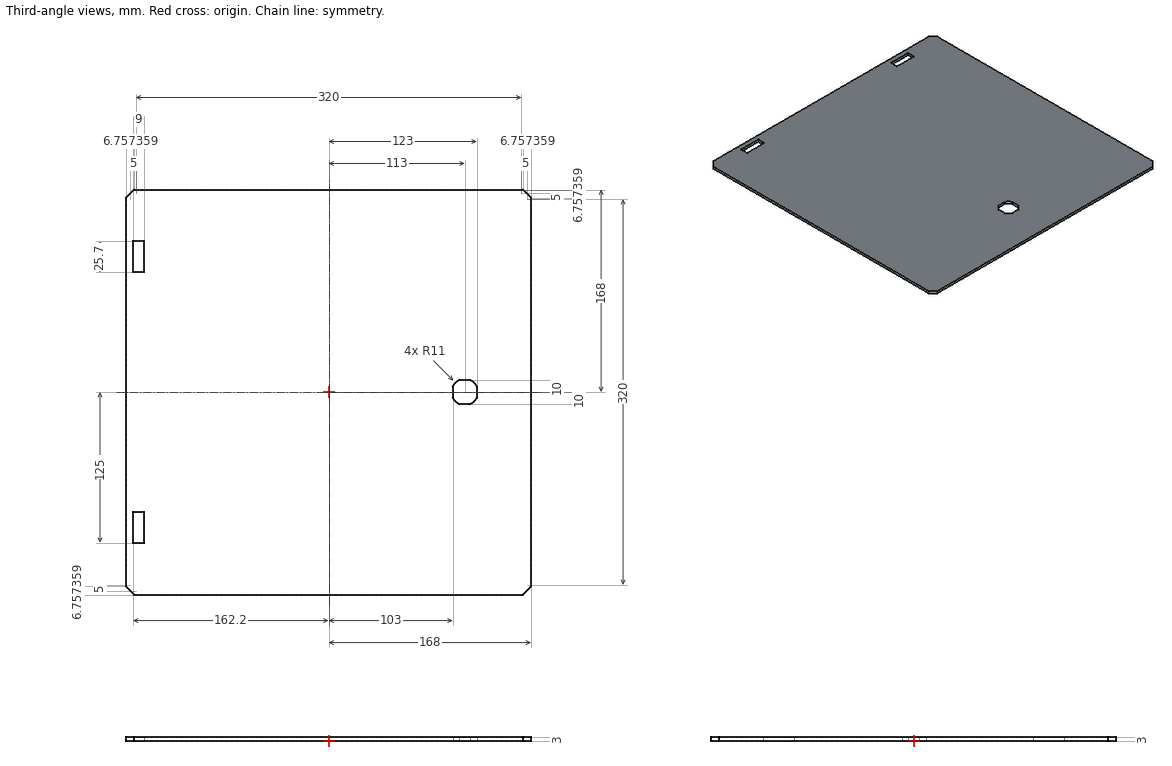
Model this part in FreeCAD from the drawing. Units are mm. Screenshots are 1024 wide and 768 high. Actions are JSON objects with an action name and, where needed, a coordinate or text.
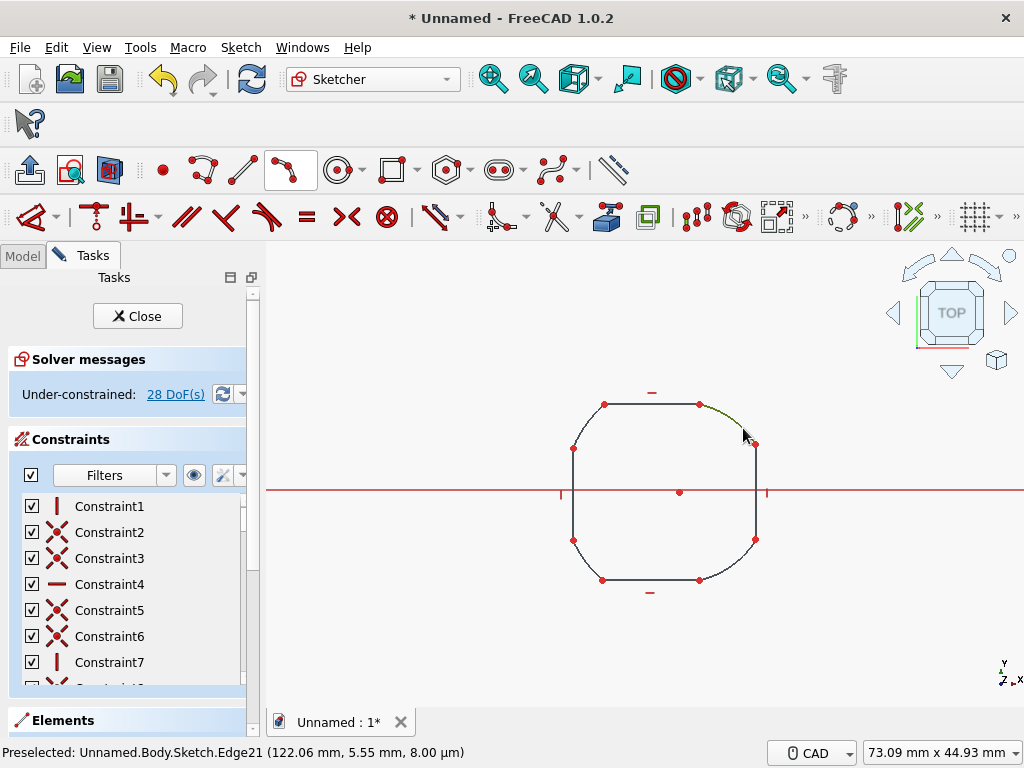
{"action": "left_click", "coordinate": [719, 573]}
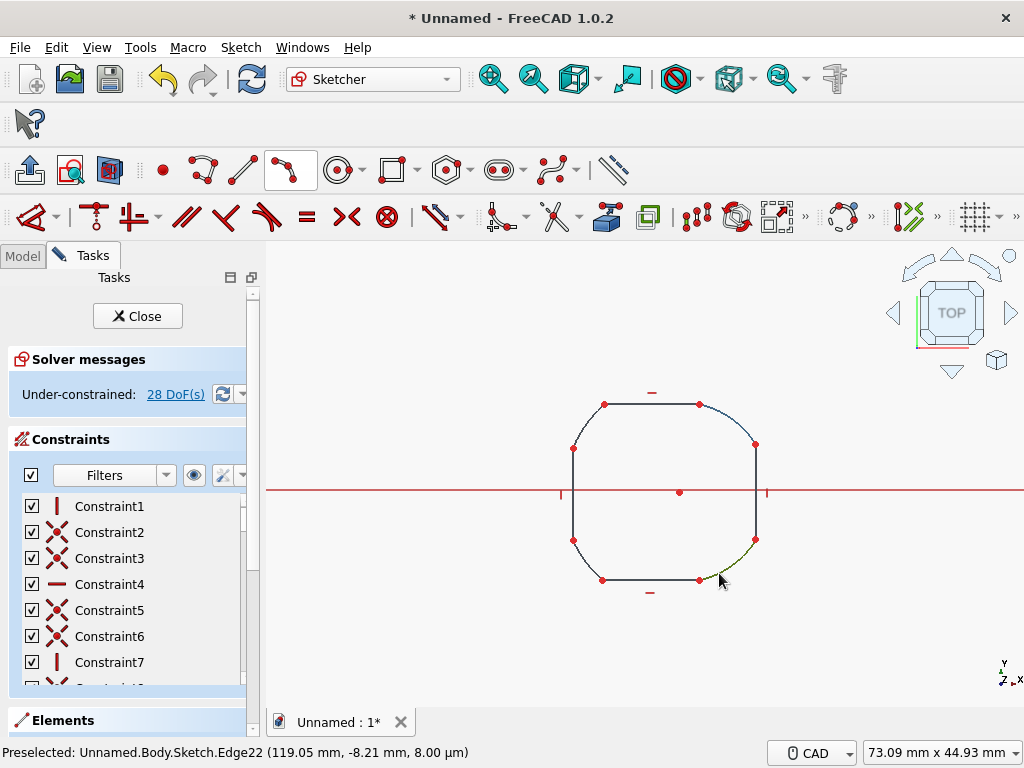
{"action": "left_click", "coordinate": [580, 554]}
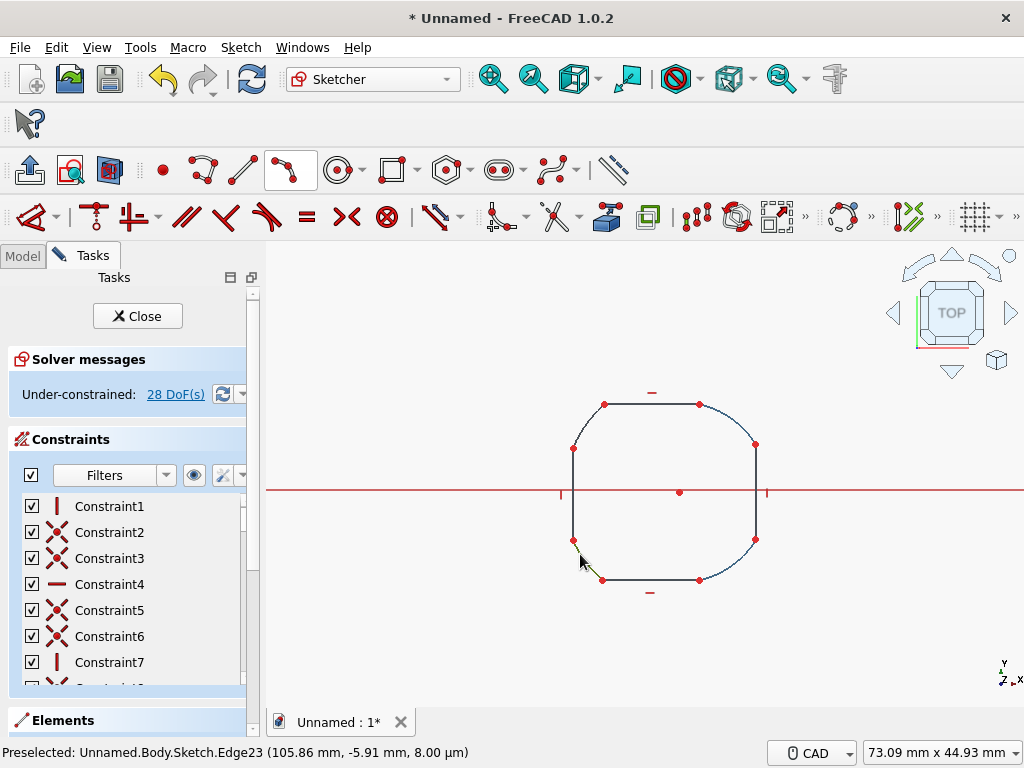
{"action": "left_click", "coordinate": [593, 416]}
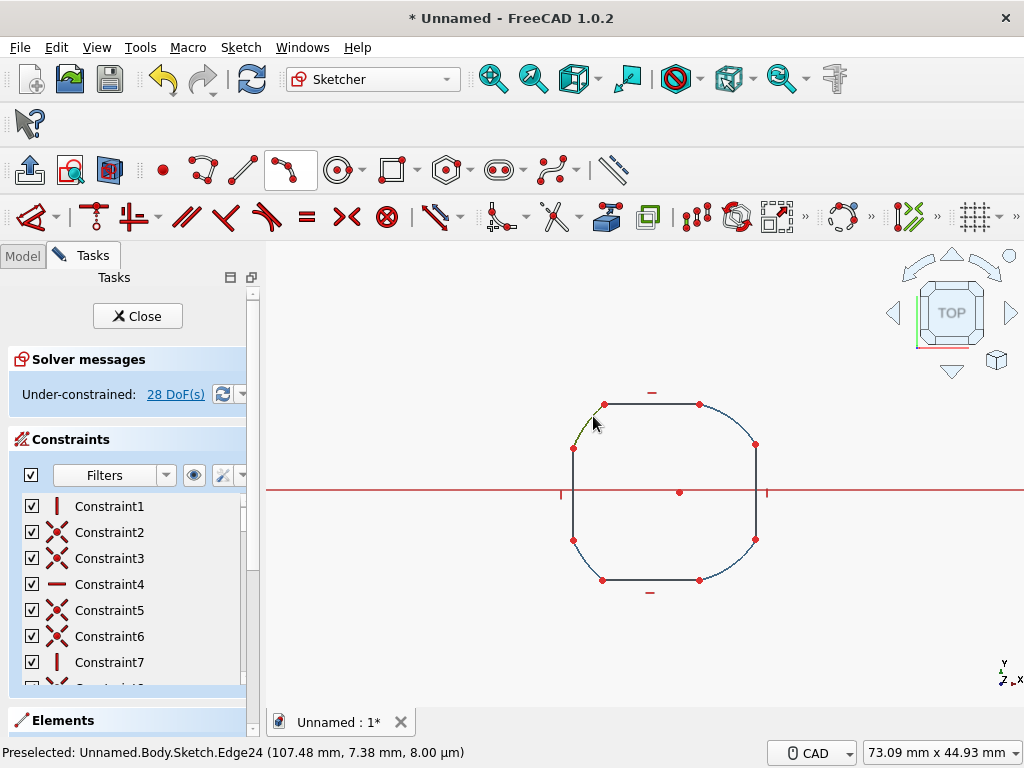
{"action": "left_click", "coordinate": [308, 218]}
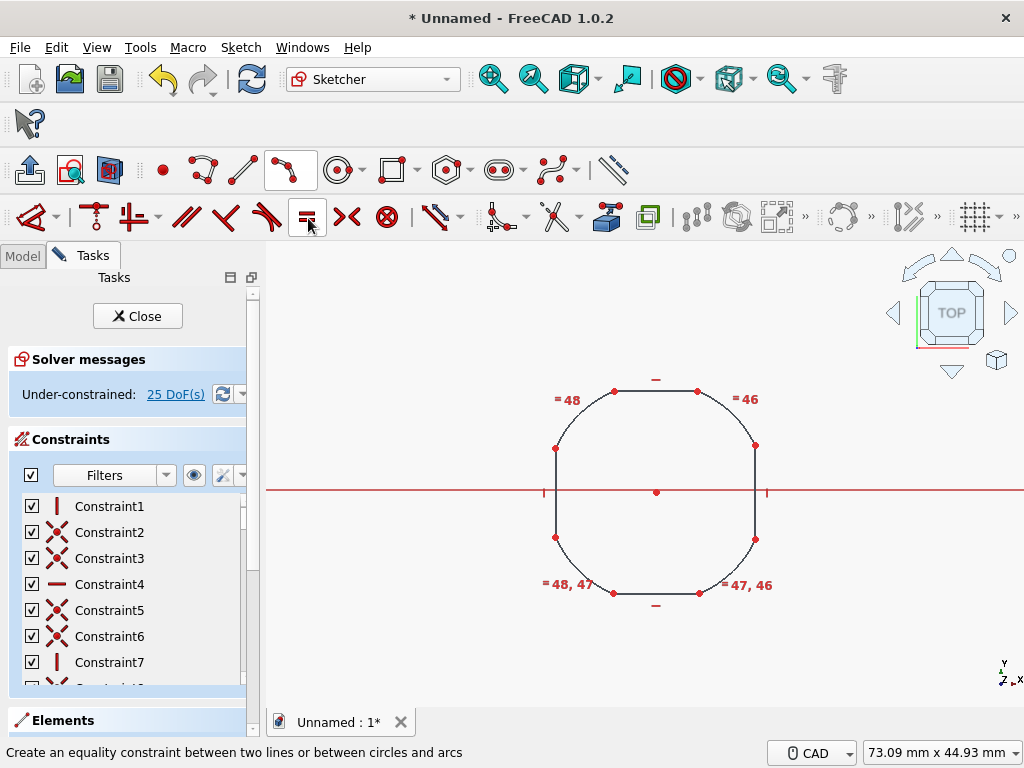
{"action": "scroll", "coordinate": [686, 472], "scroll_direction": "down", "scroll_amount": 12}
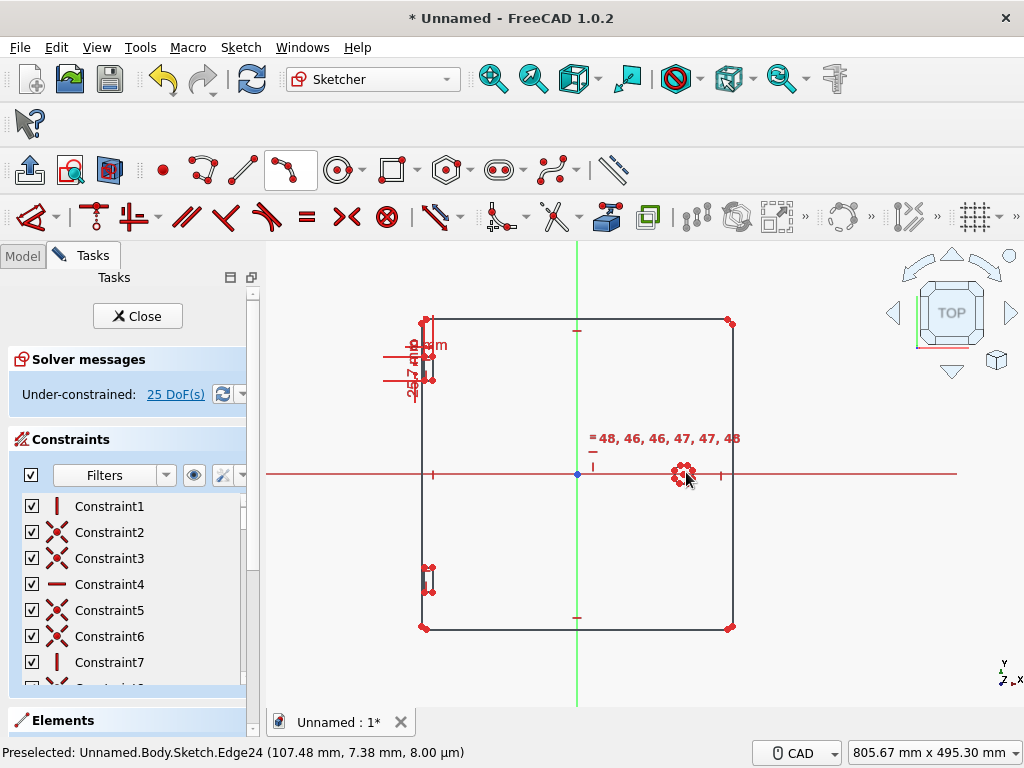
{"action": "scroll", "coordinate": [684, 474], "scroll_direction": "up", "scroll_amount": 2}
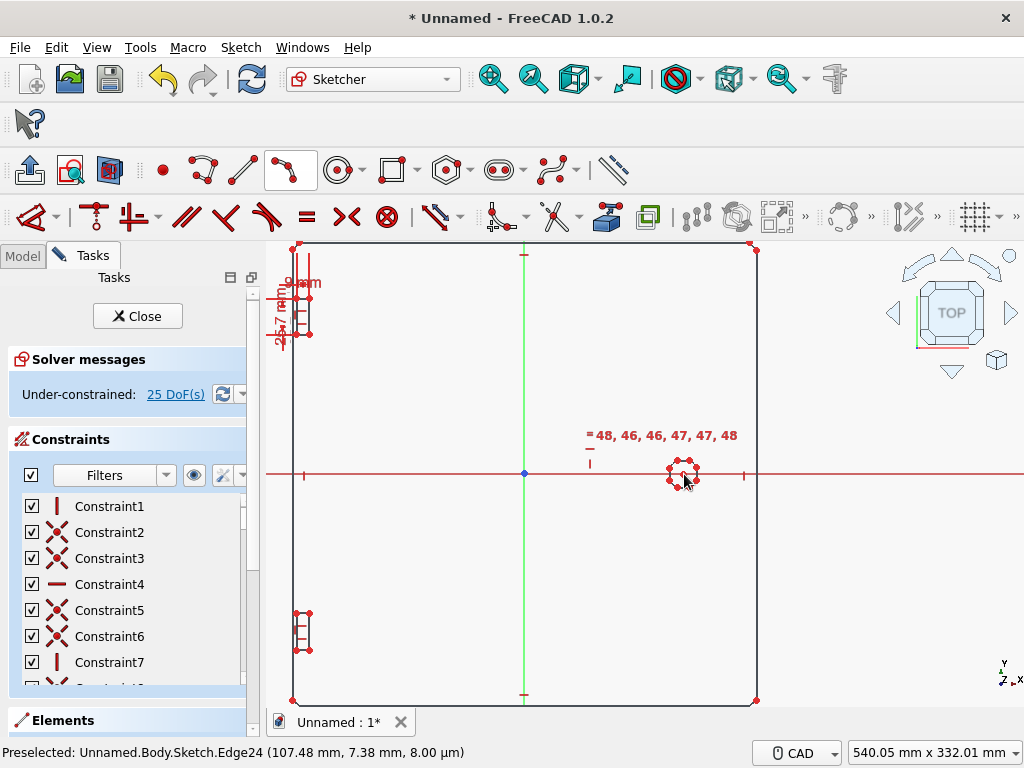
{"action": "left_click", "coordinate": [683, 474]}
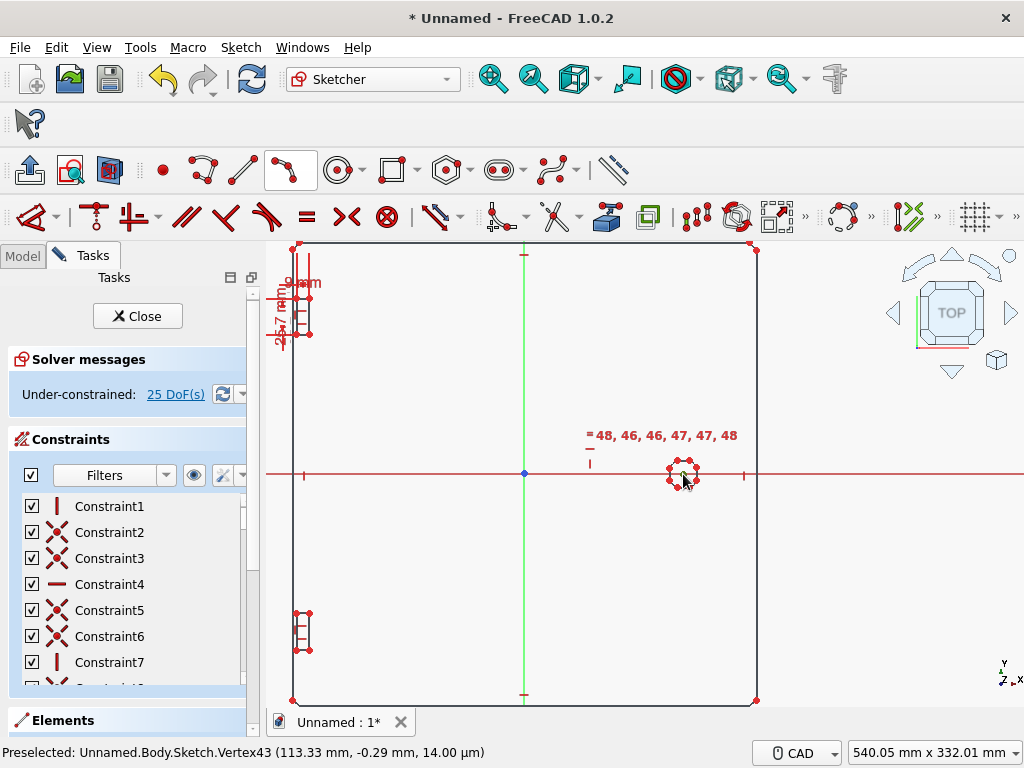
{"action": "left_click", "coordinate": [334, 474]}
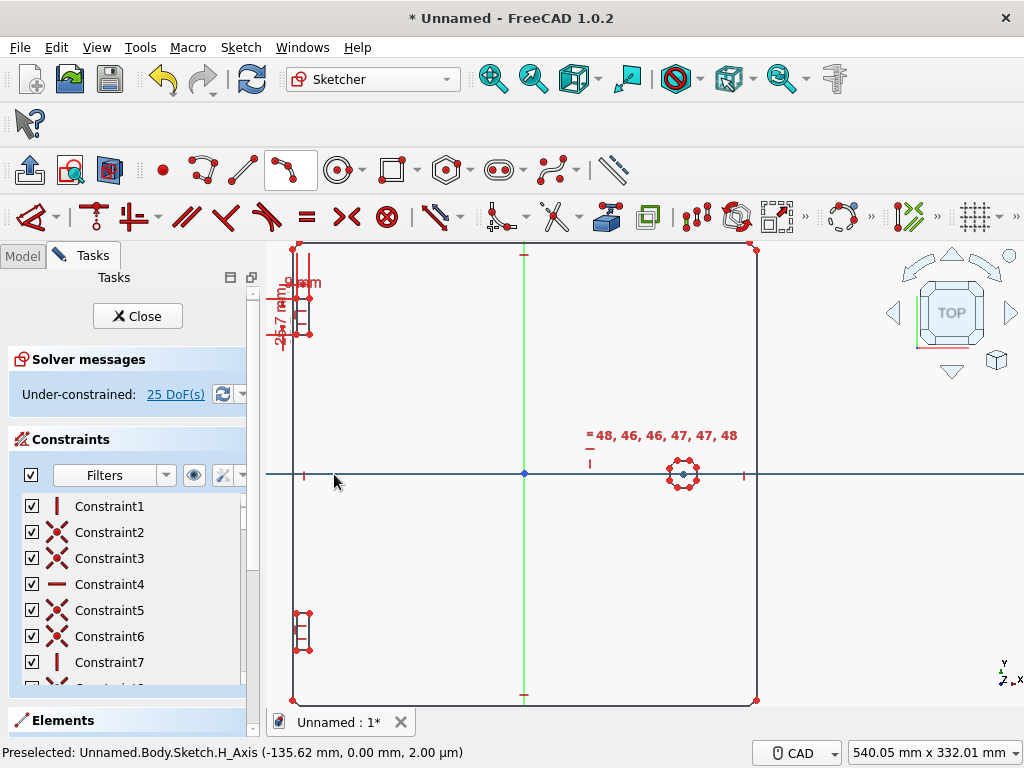
{"action": "left_click", "coordinate": [94, 218]}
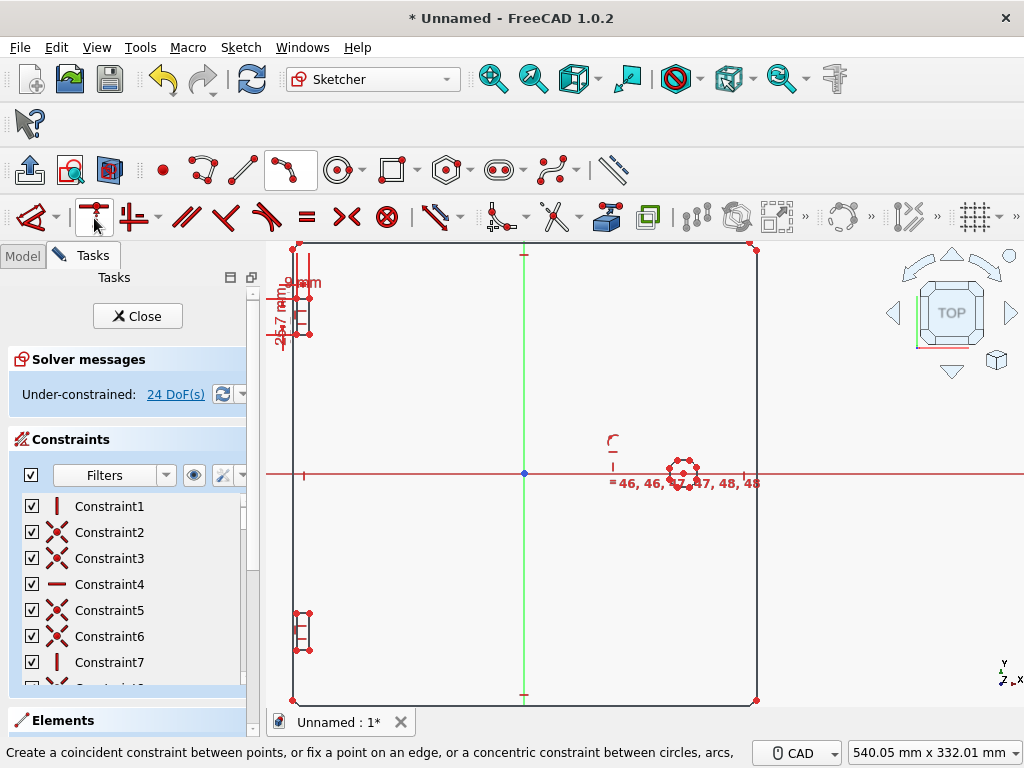
{"action": "scroll", "coordinate": [683, 474], "scroll_direction": "down", "scroll_amount": 2}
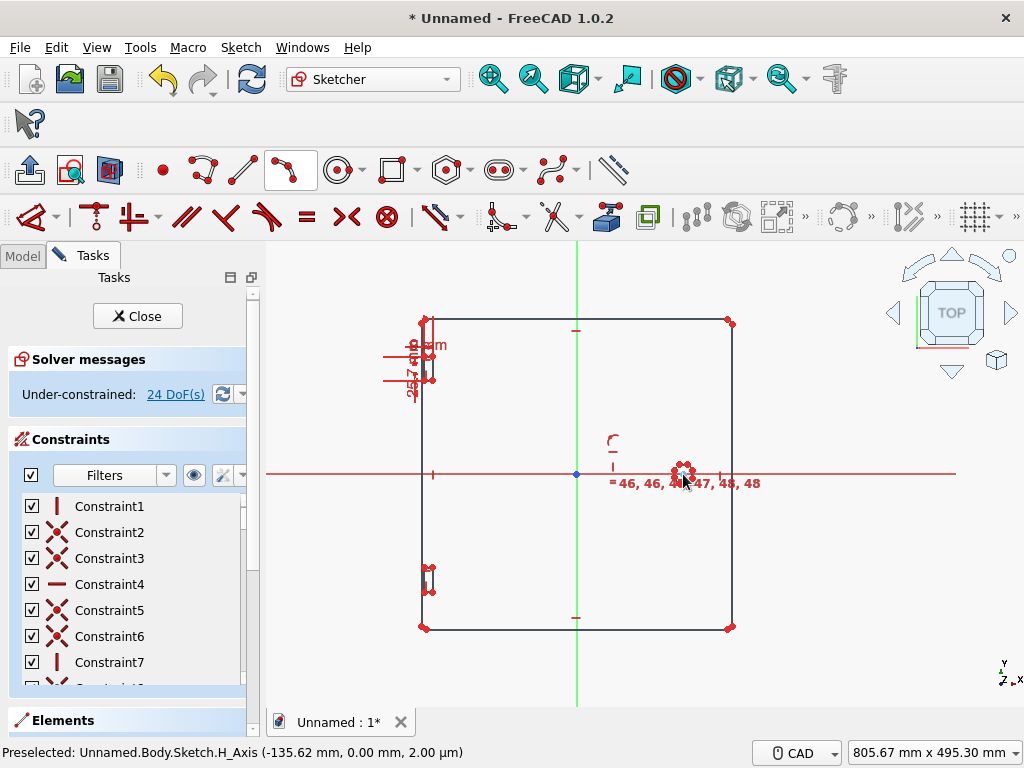
{"action": "scroll", "coordinate": [732, 324], "scroll_direction": "up", "scroll_amount": 3}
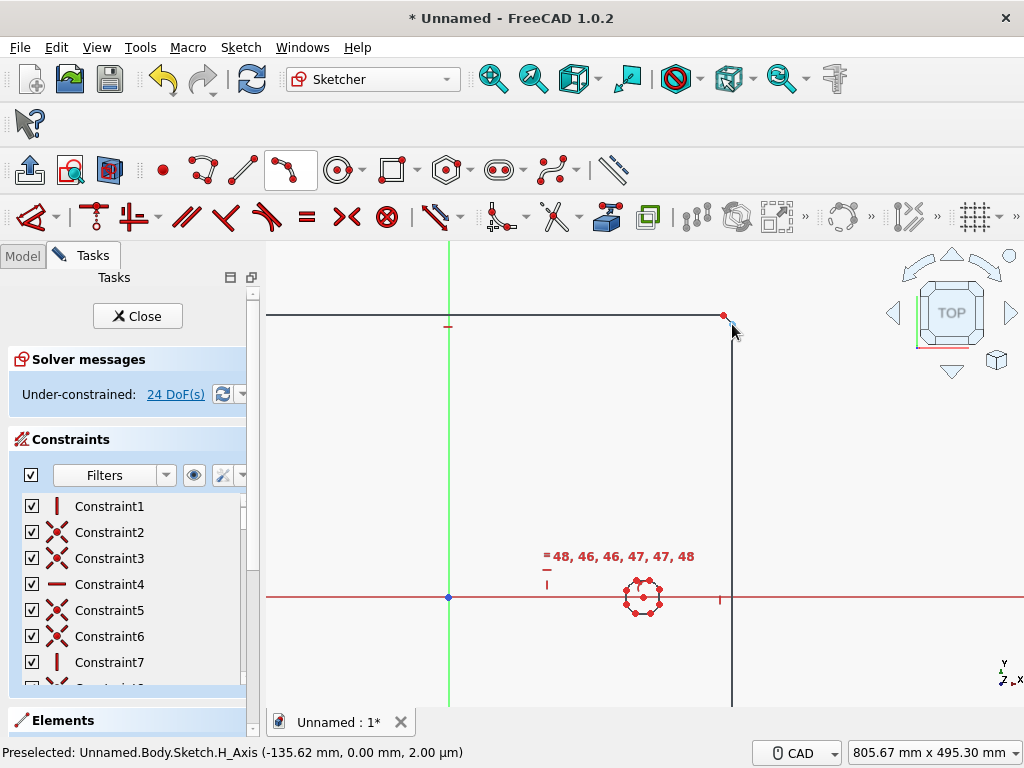
{"action": "left_click", "coordinate": [732, 324]}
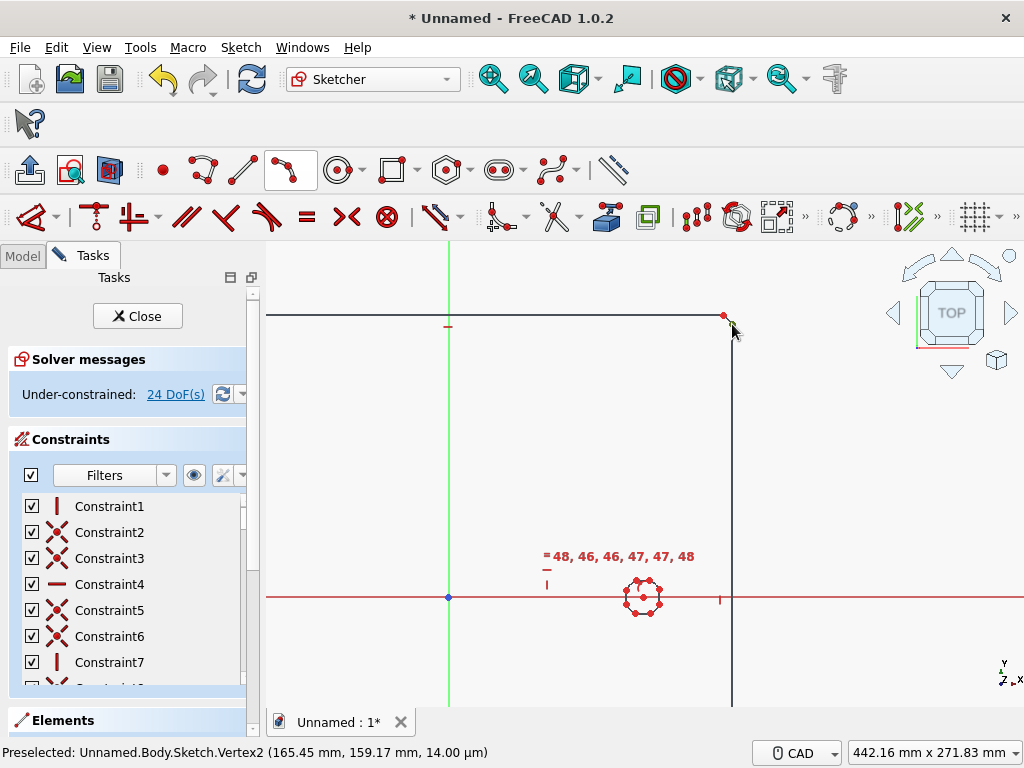
{"action": "scroll", "coordinate": [732, 324], "scroll_direction": "down", "scroll_amount": 3}